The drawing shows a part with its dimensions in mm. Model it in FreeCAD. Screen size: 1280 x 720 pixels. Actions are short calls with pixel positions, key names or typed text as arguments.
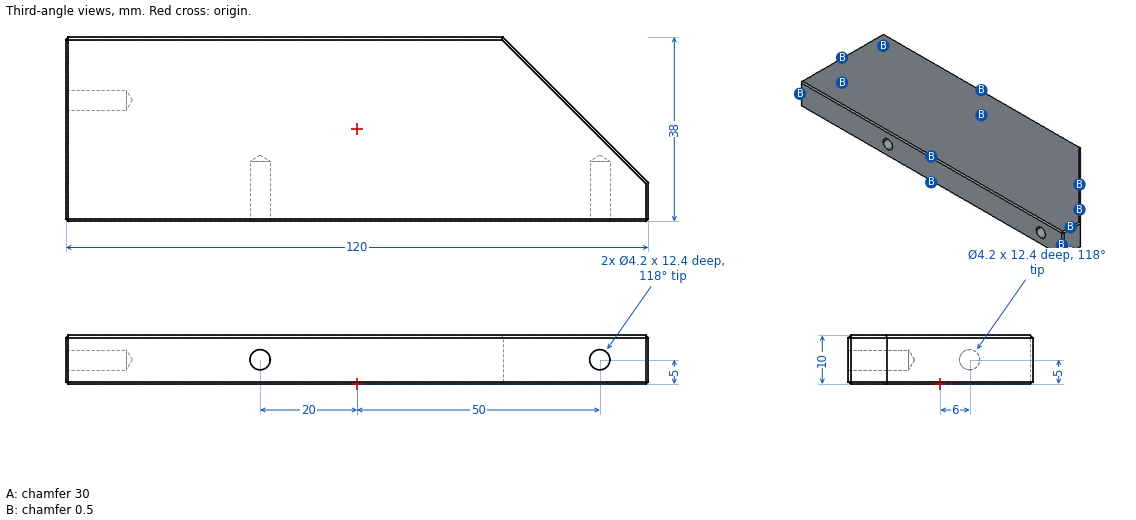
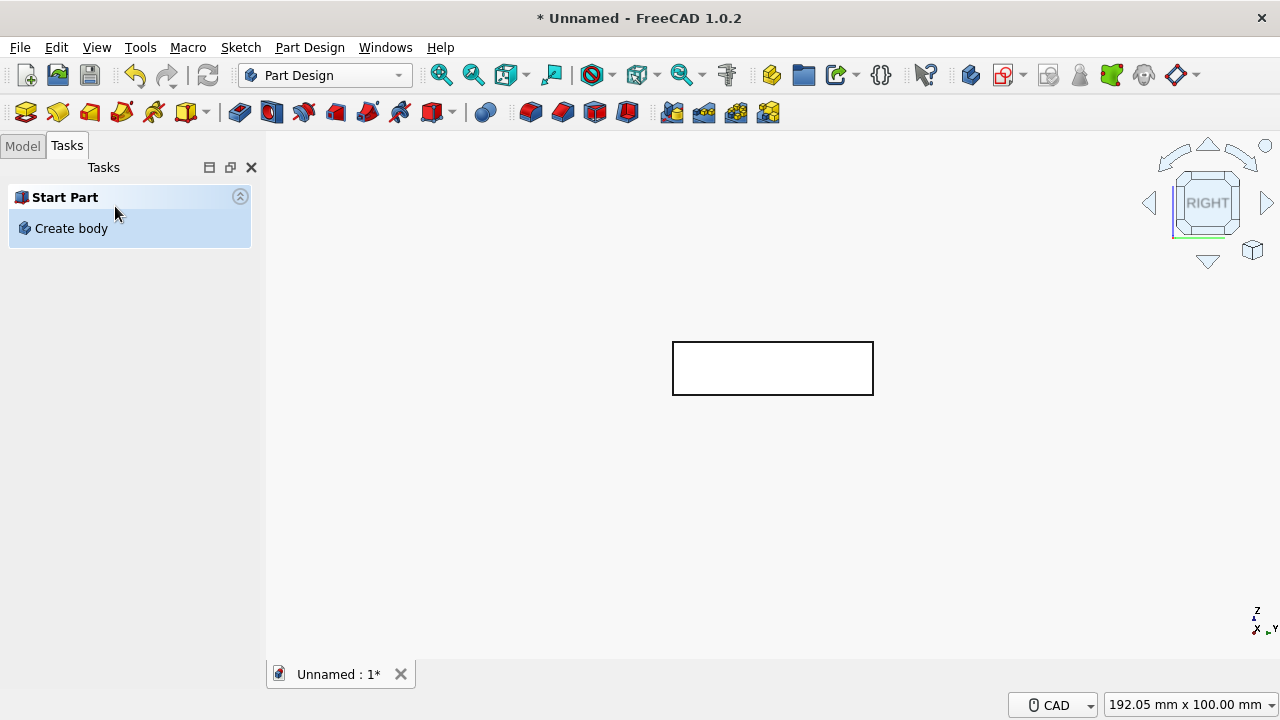
click(442, 76)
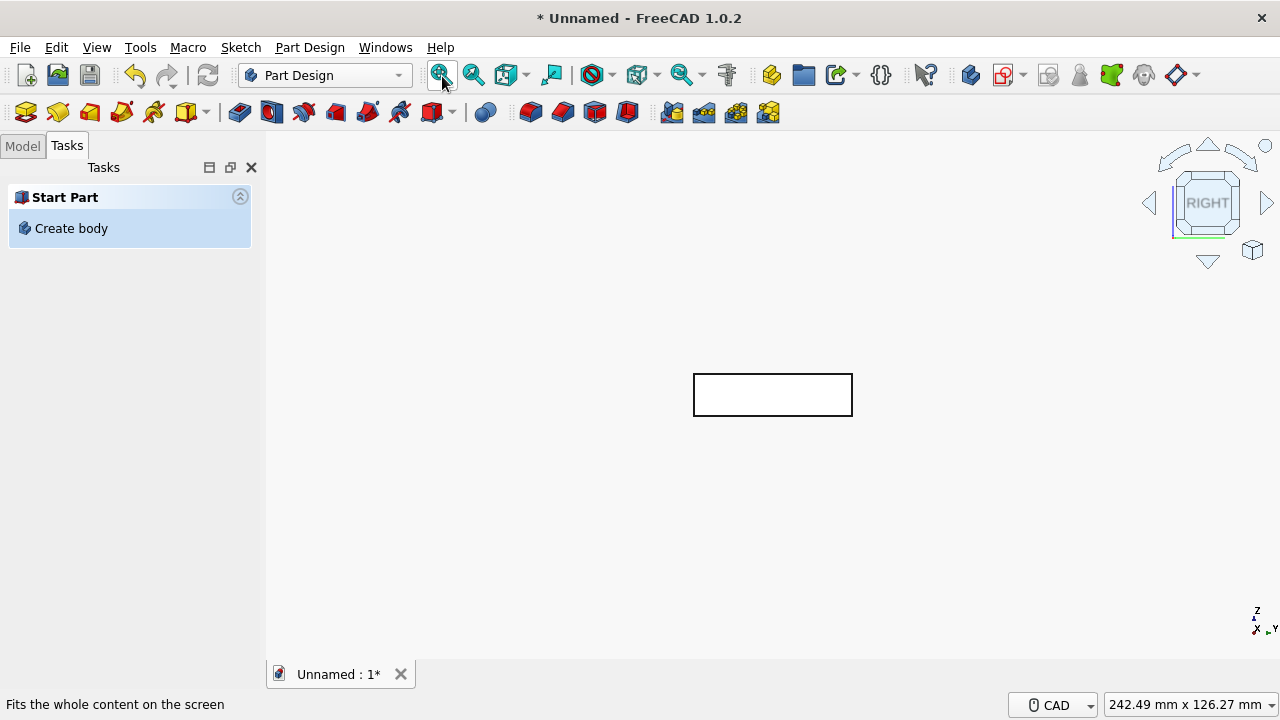
click(852, 394)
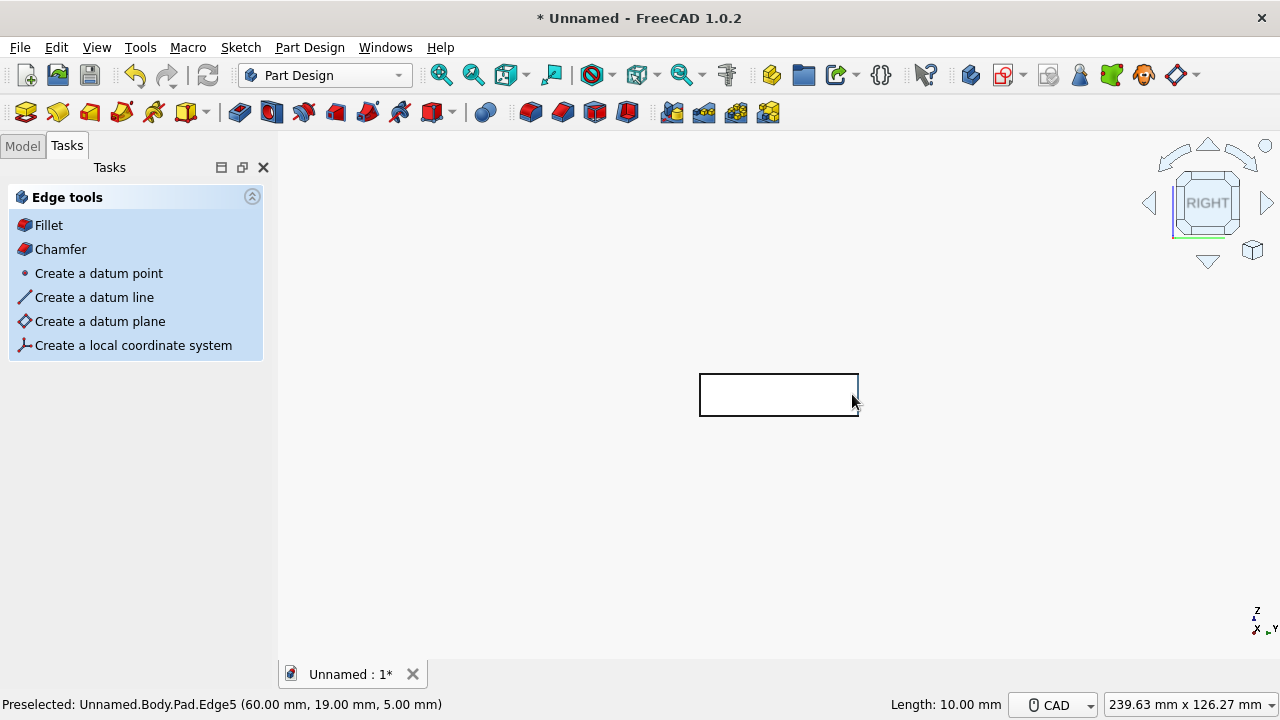
click(564, 112)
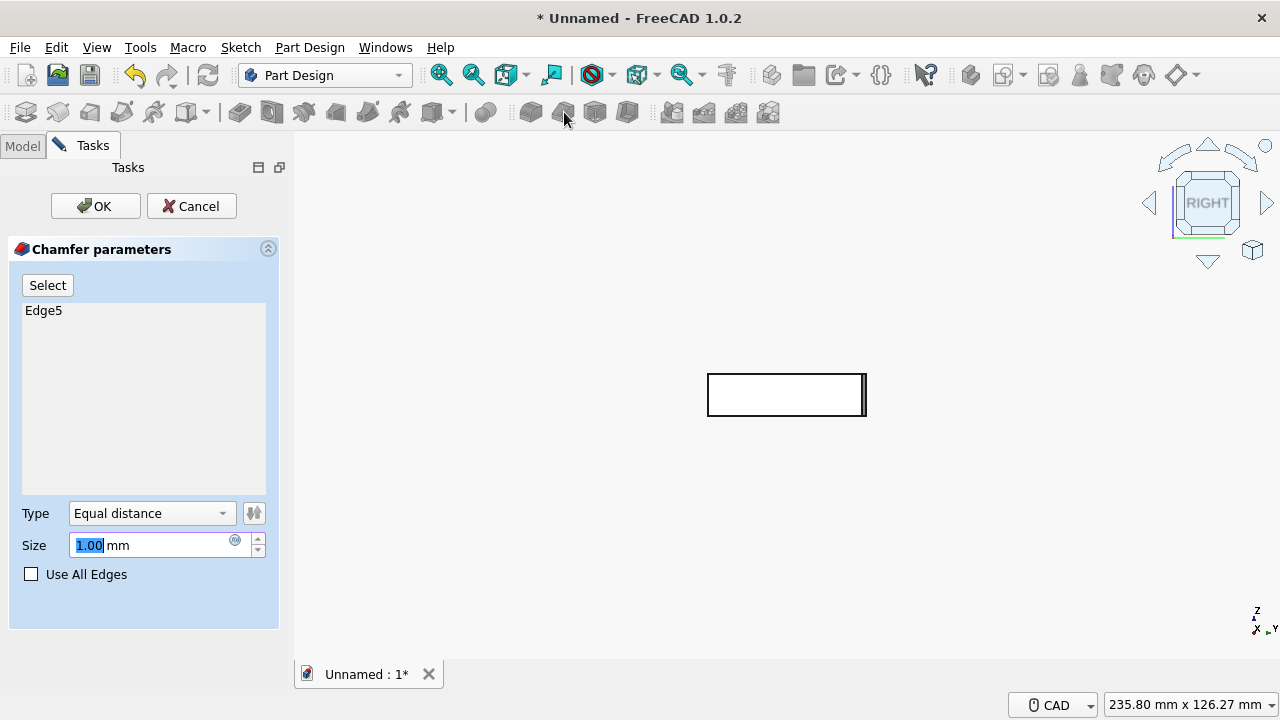
text(30)
key(Tab)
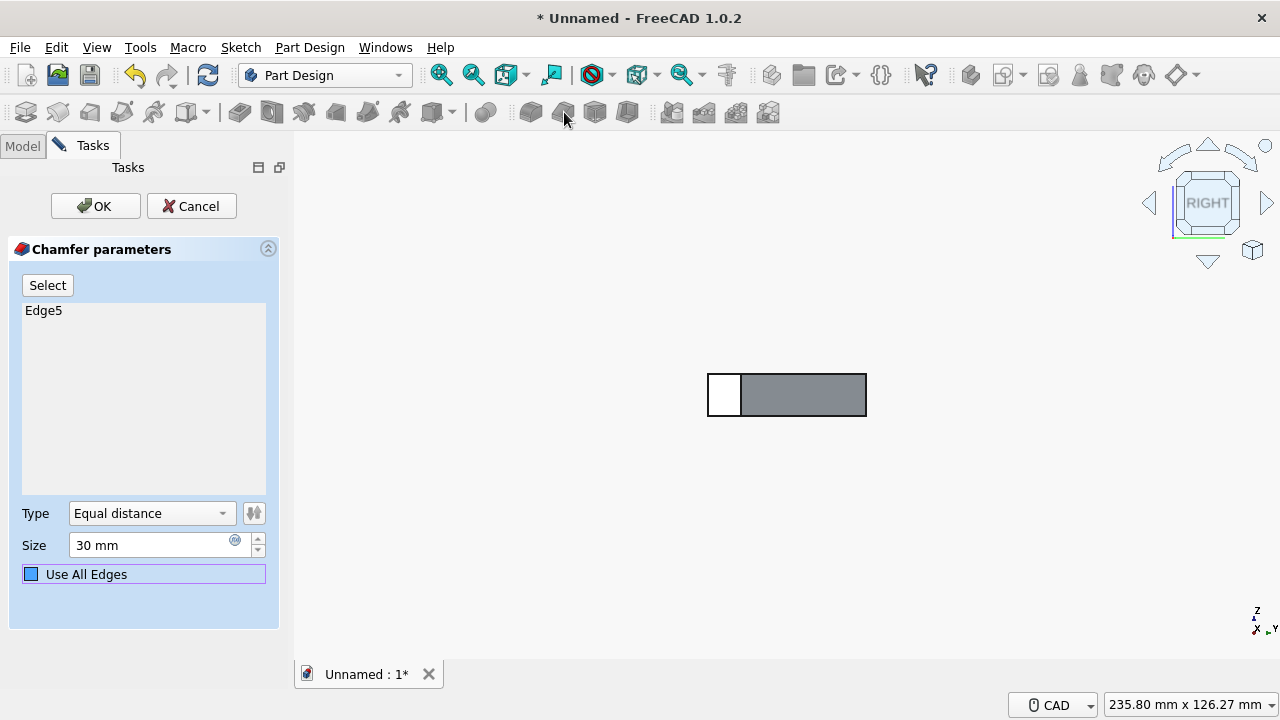
click(96, 206)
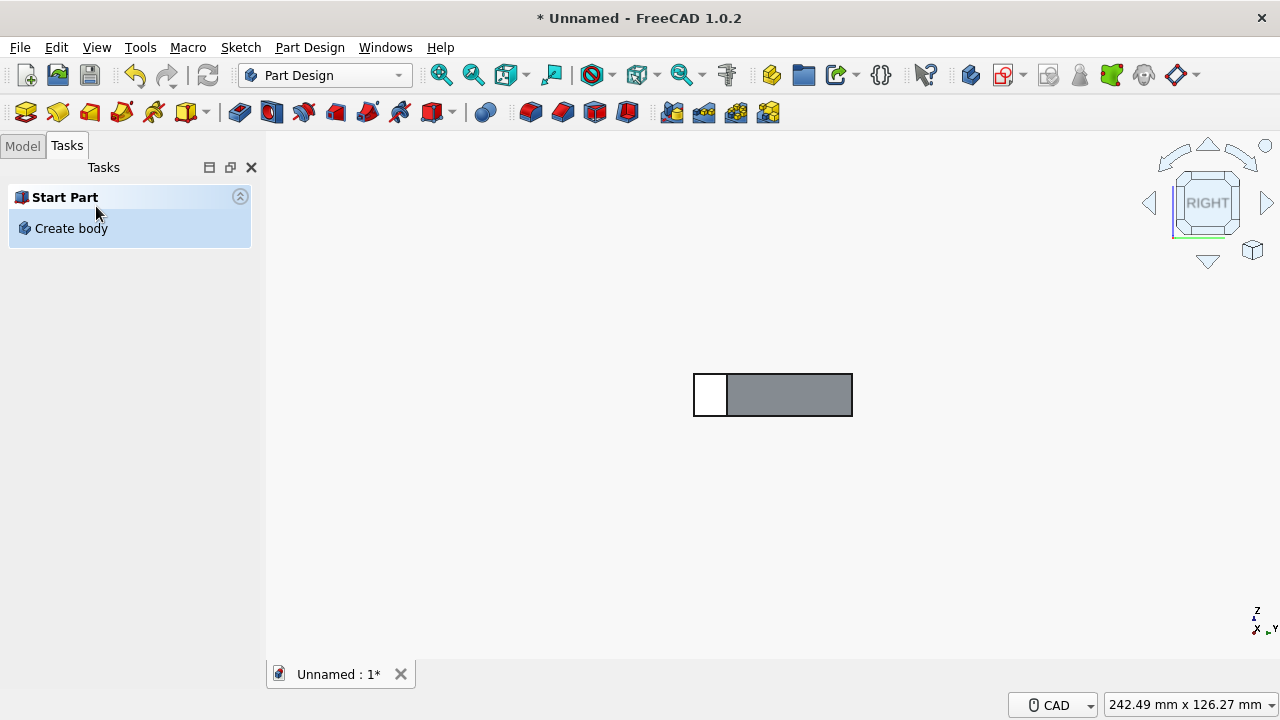
click(442, 76)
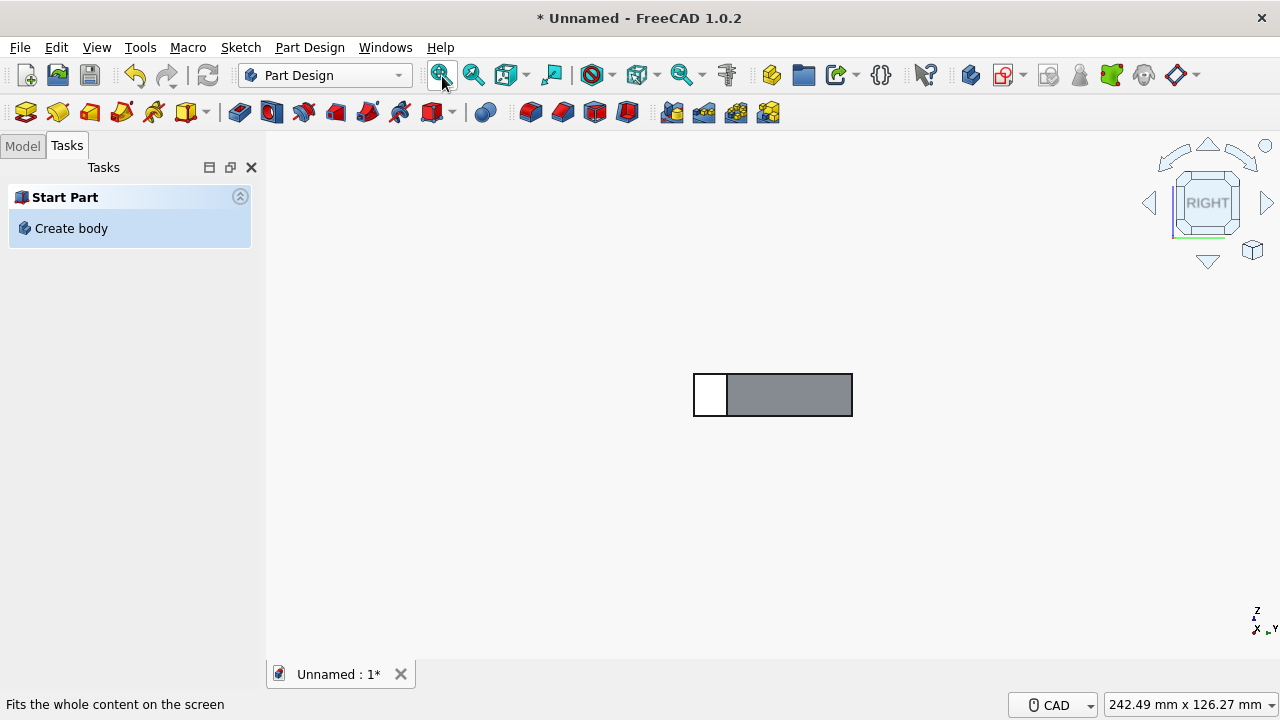
key(6)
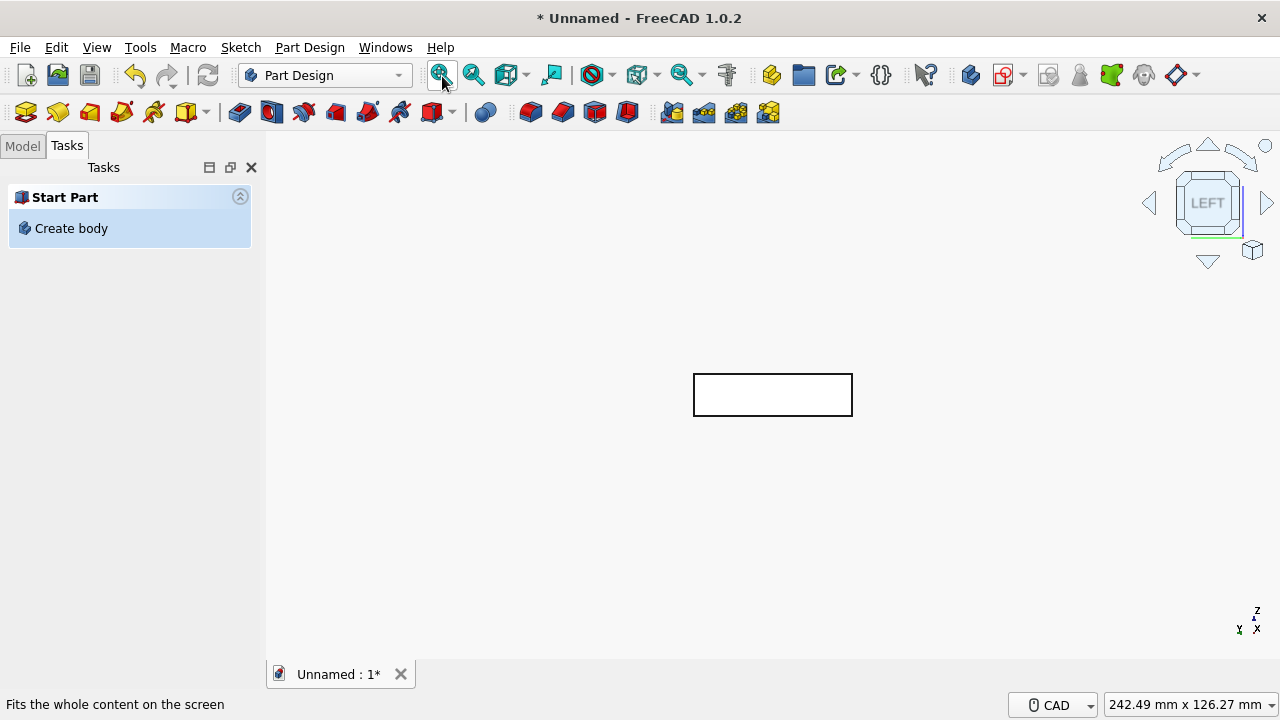
click(442, 76)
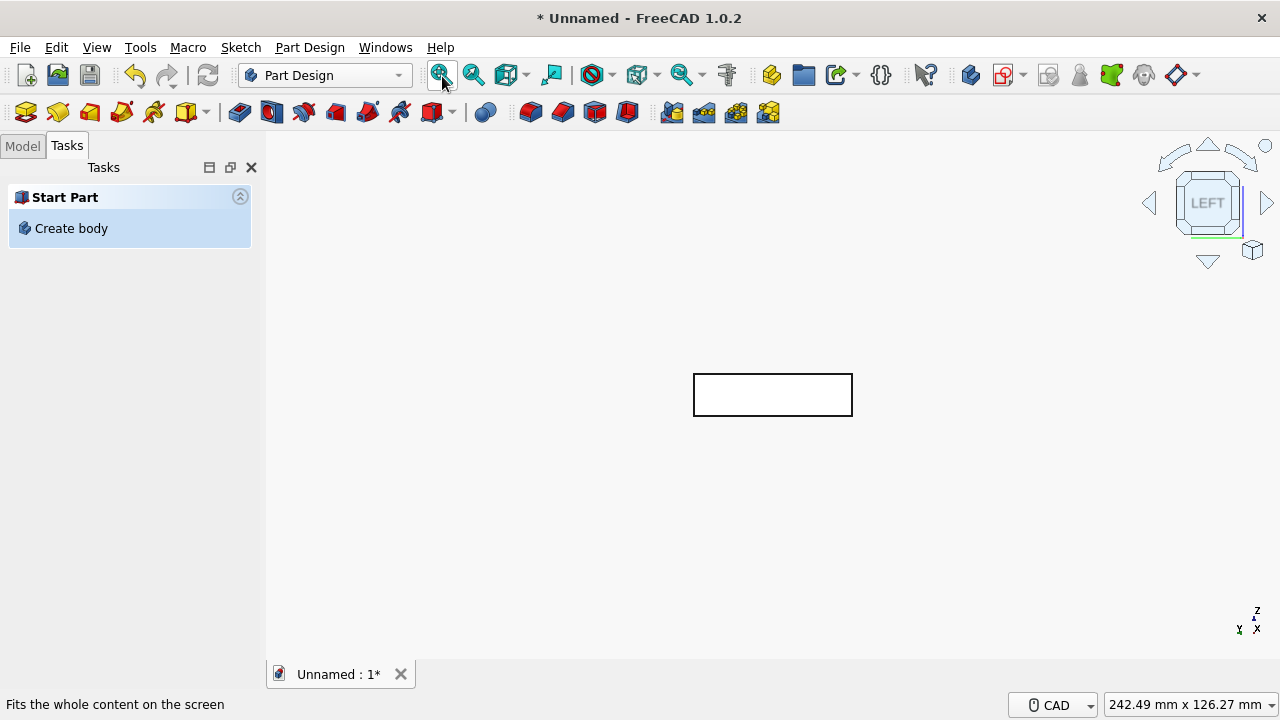
click(728, 394)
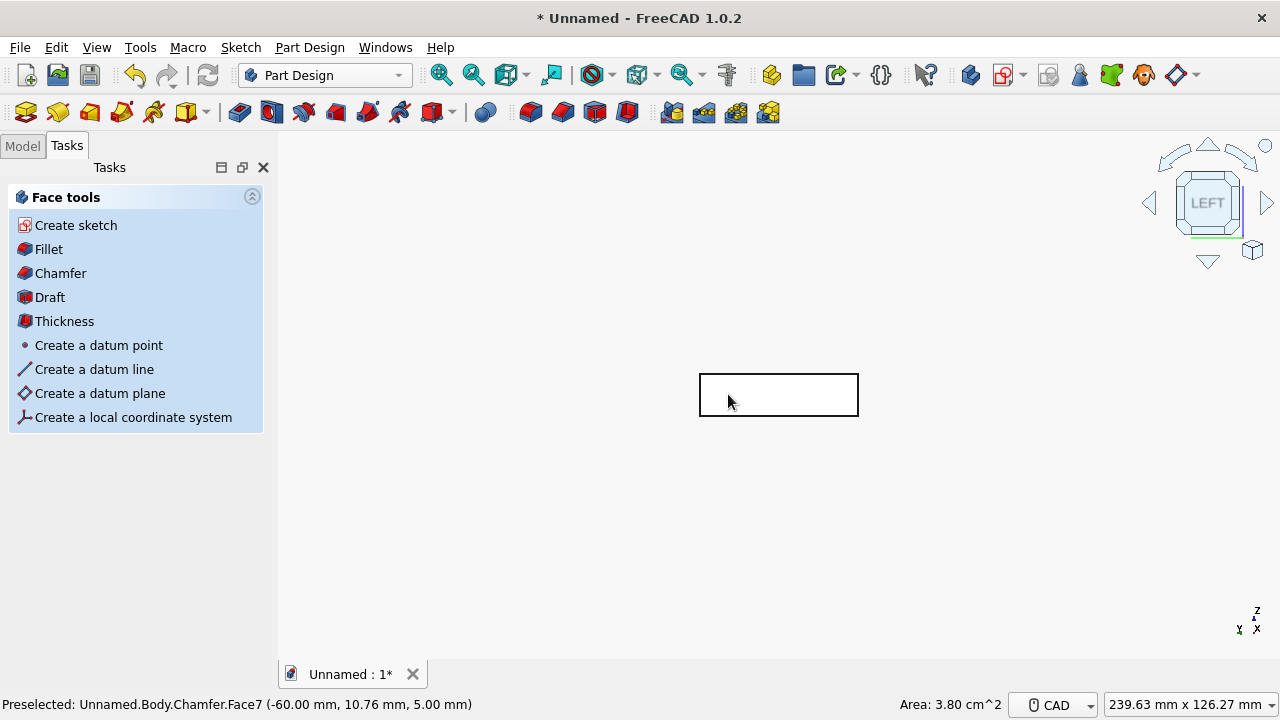
click(1004, 76)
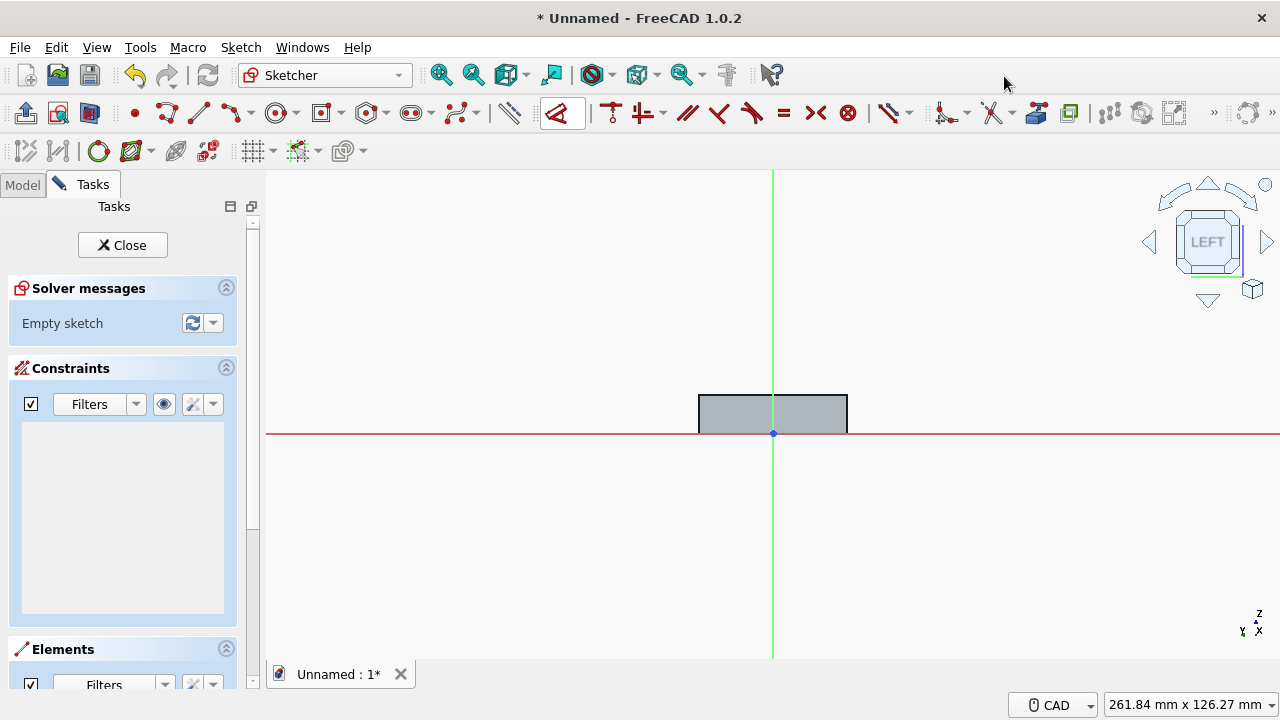
scroll(763, 421, up, 12)